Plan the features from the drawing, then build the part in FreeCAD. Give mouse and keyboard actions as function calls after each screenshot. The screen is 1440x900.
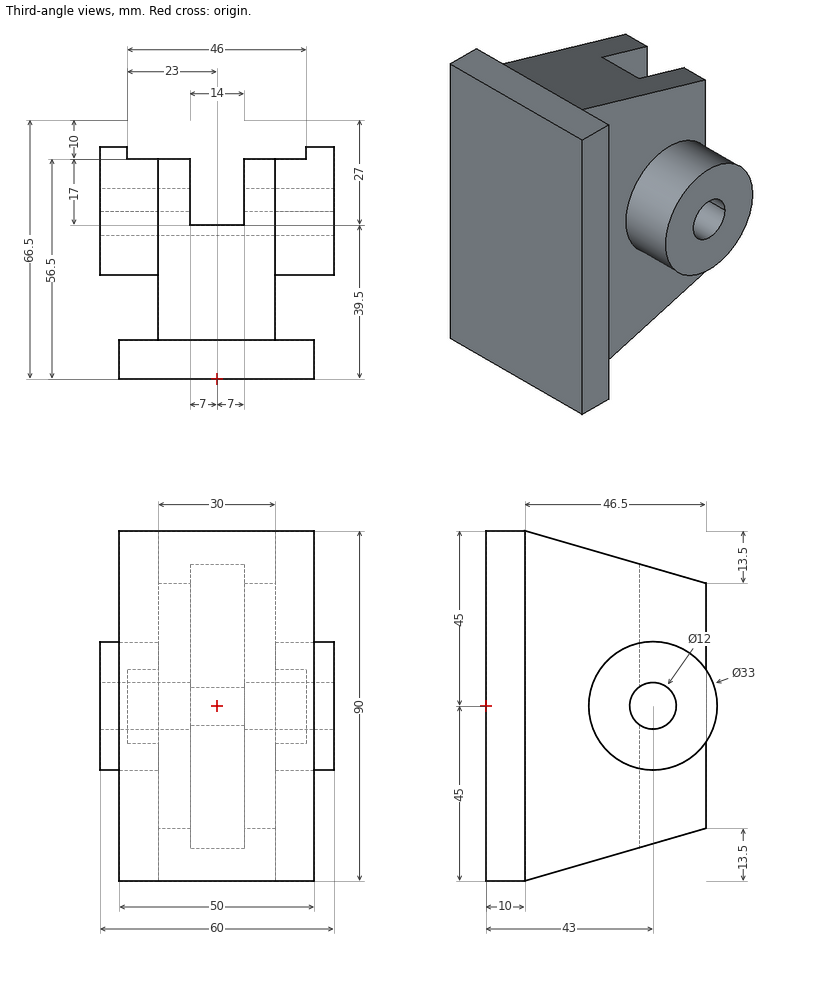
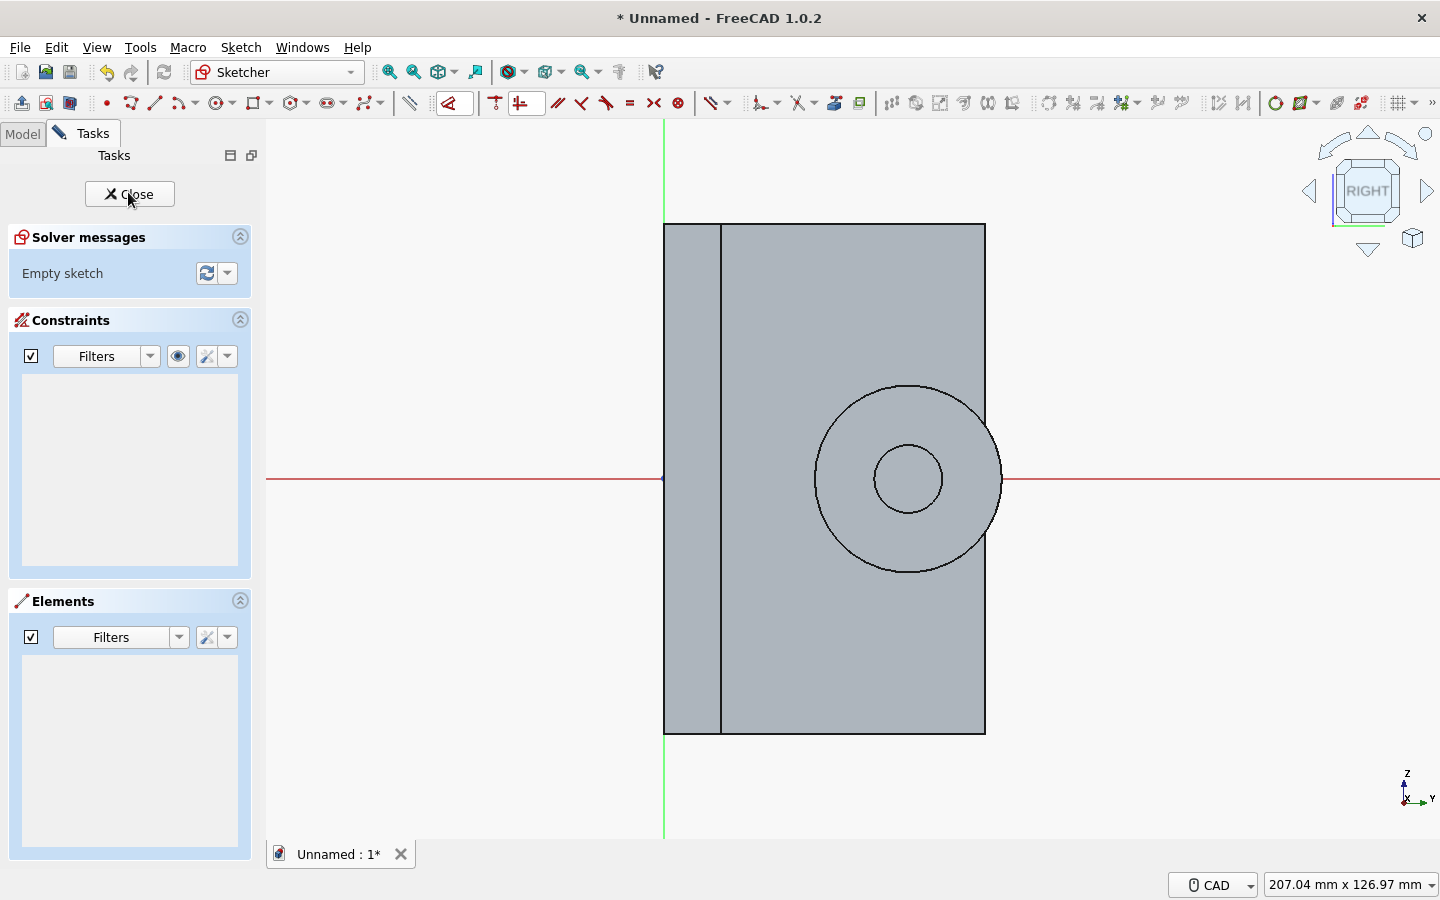
click(70, 104)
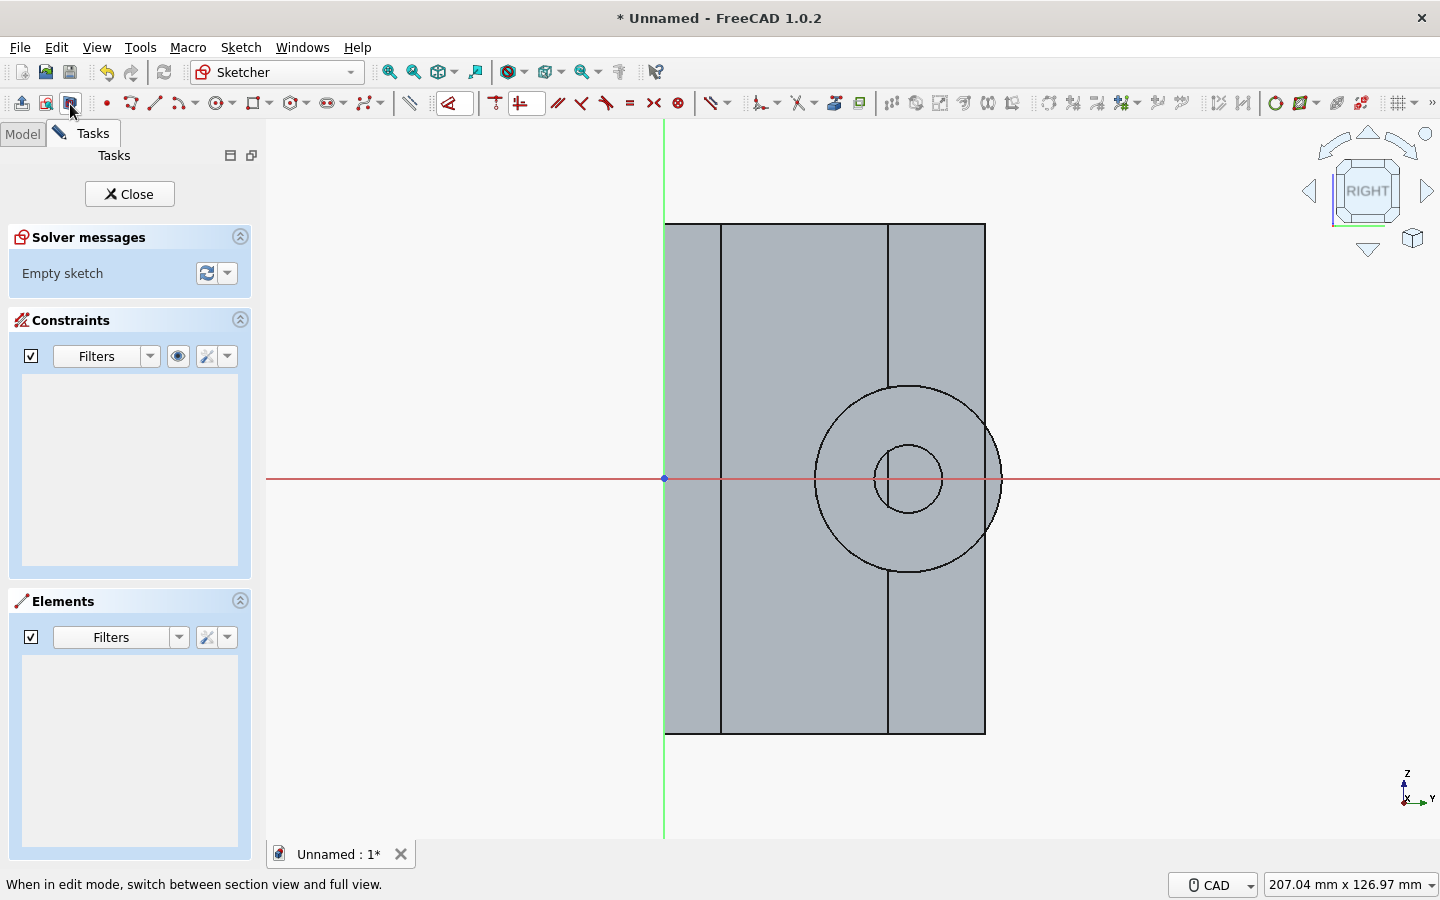
click(132, 104)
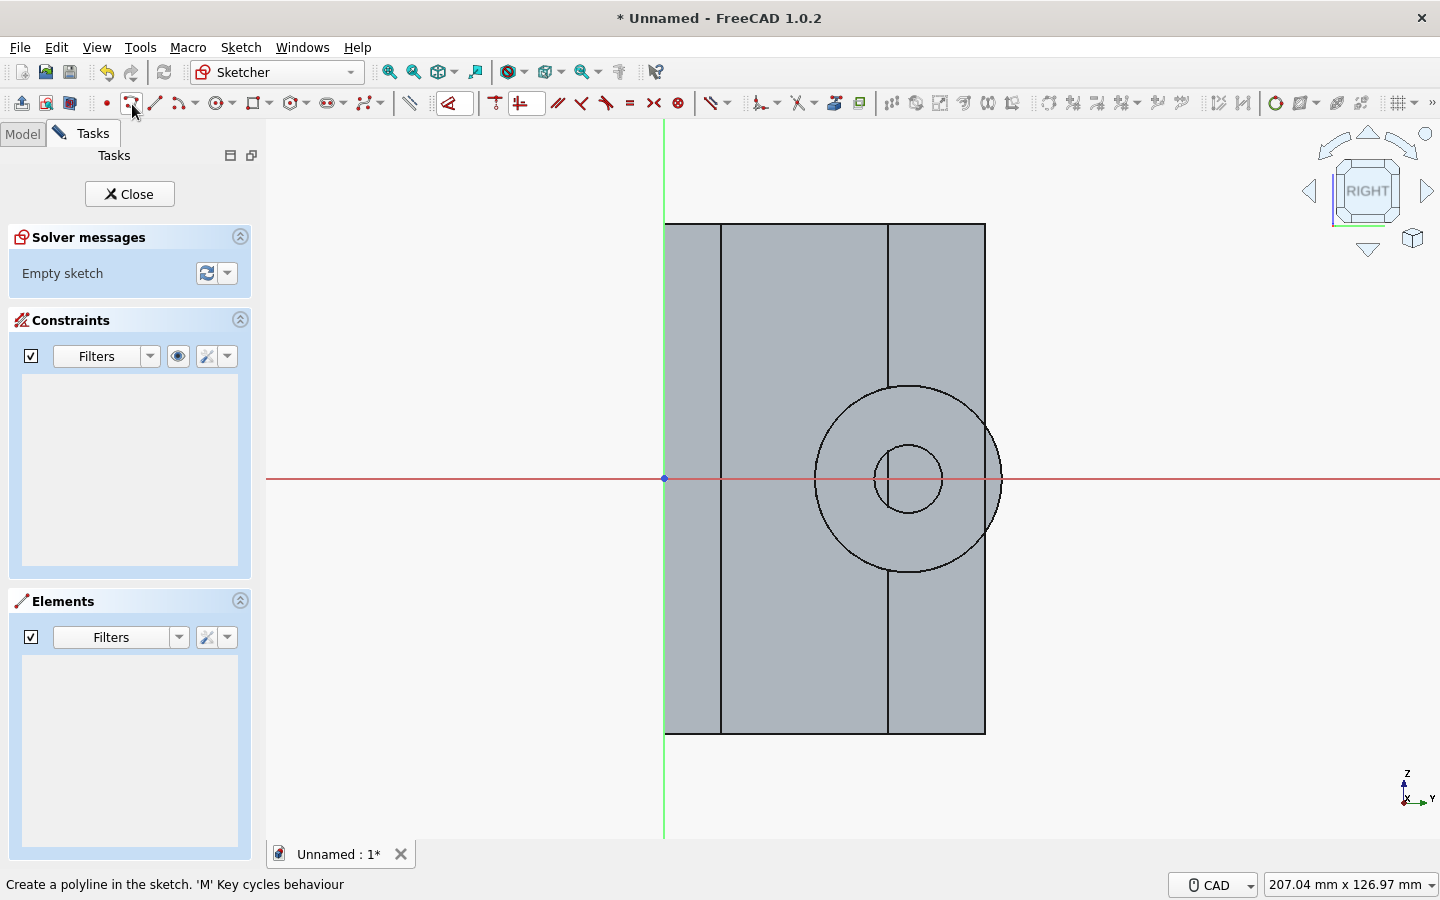
click(721, 224)
click(985, 300)
click(985, 224)
click(721, 225)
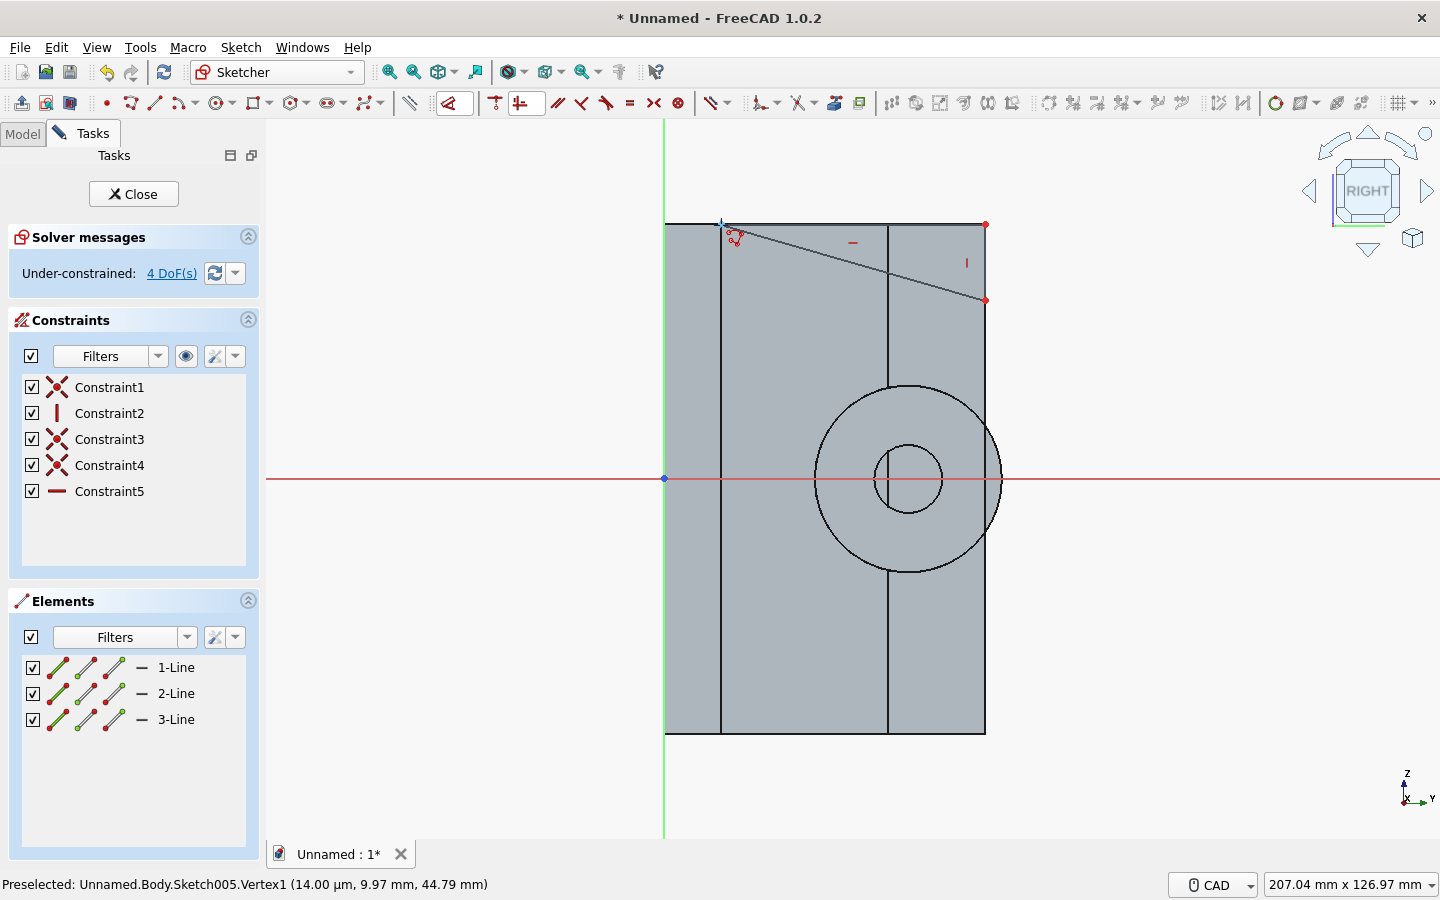
click(721, 734)
click(985, 734)
click(985, 658)
click(721, 735)
key(Escape)
key(Escape)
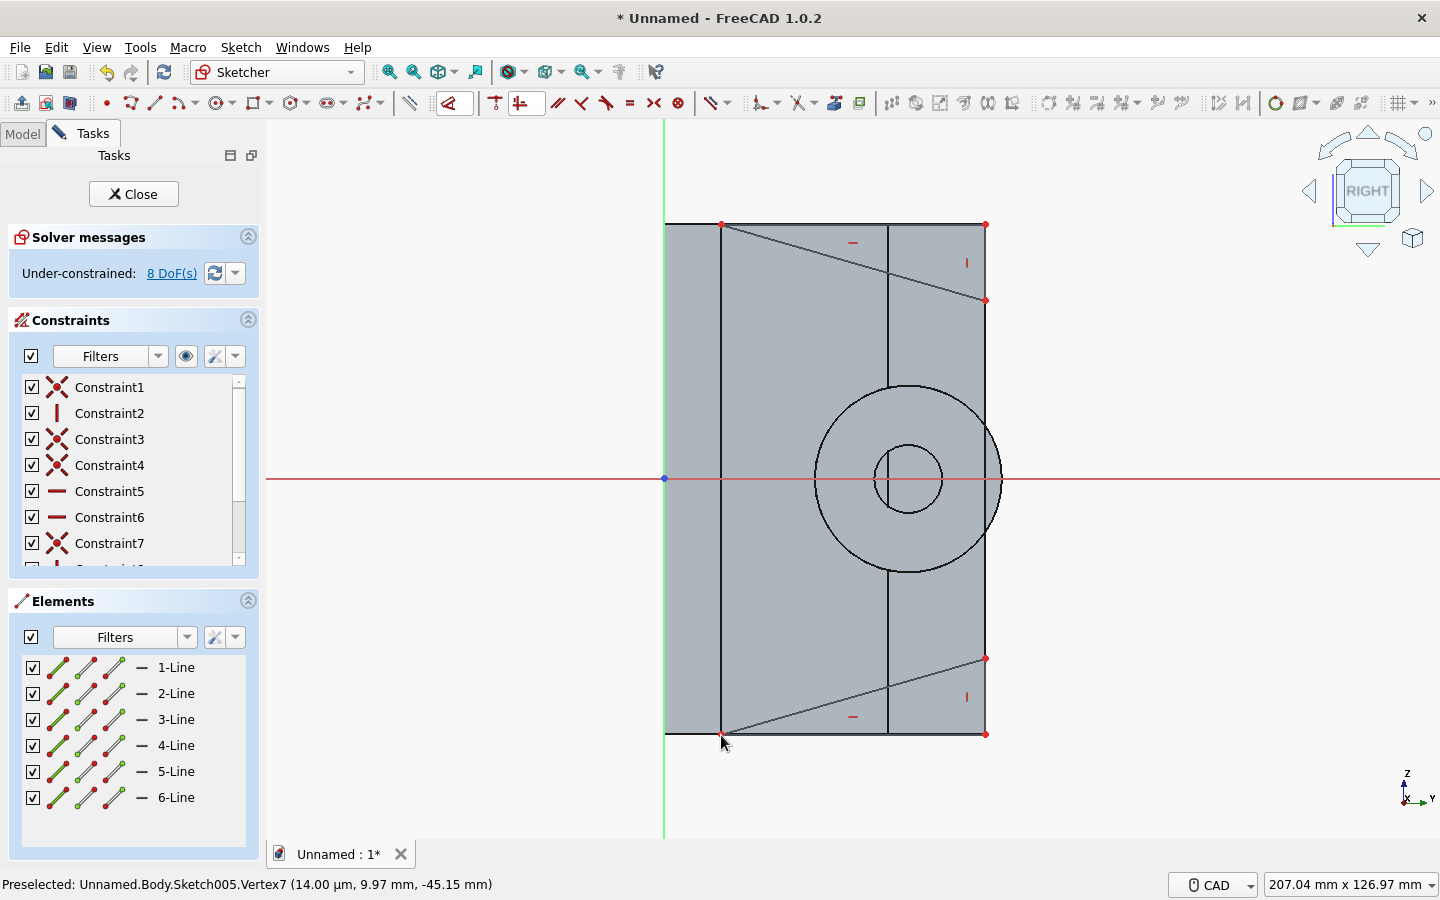
click(721, 225)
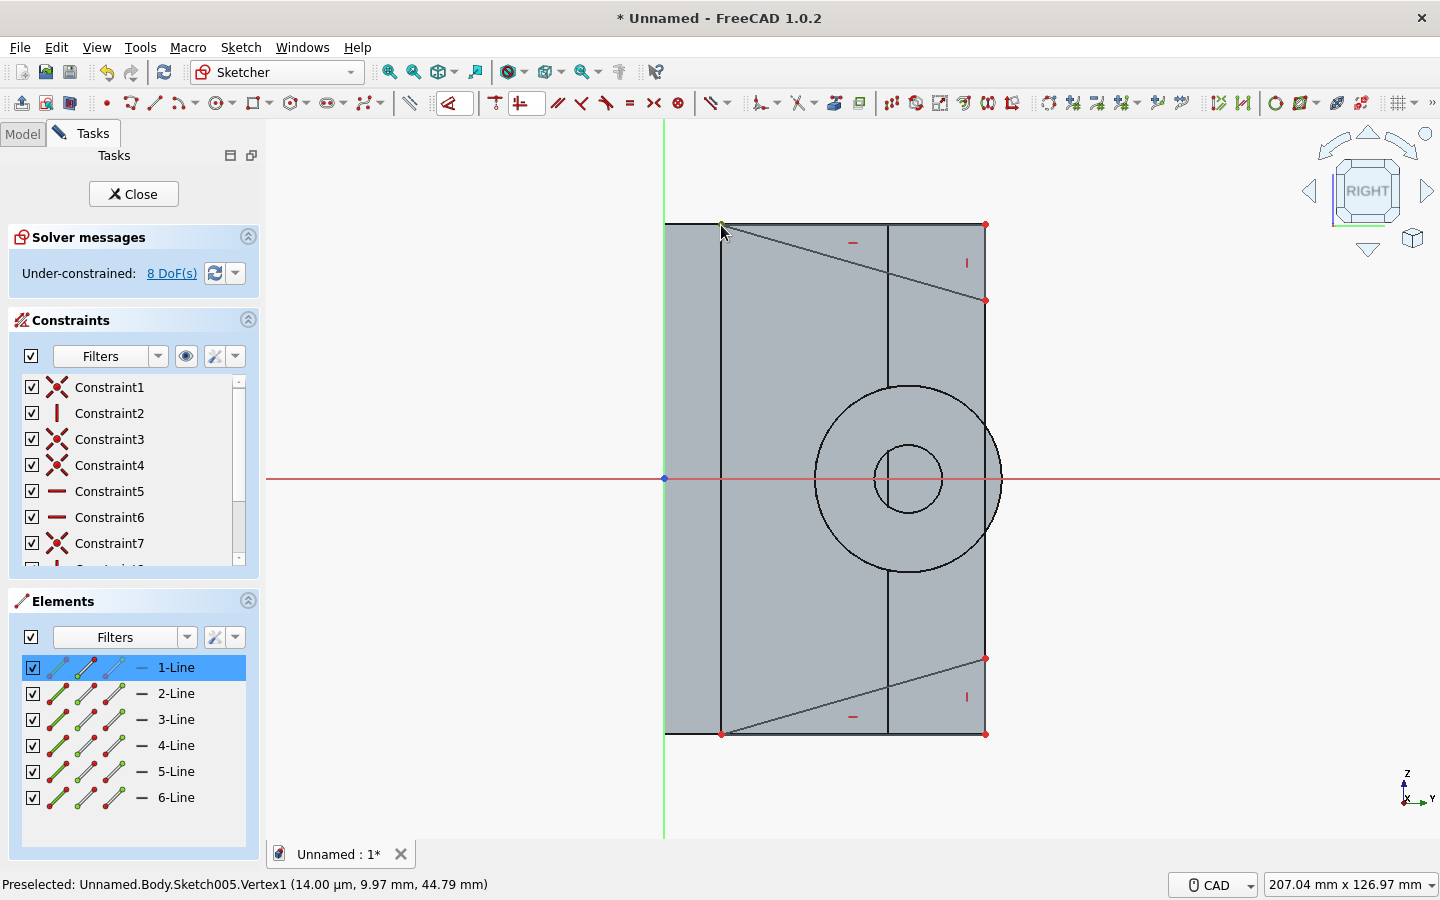
click(468, 104)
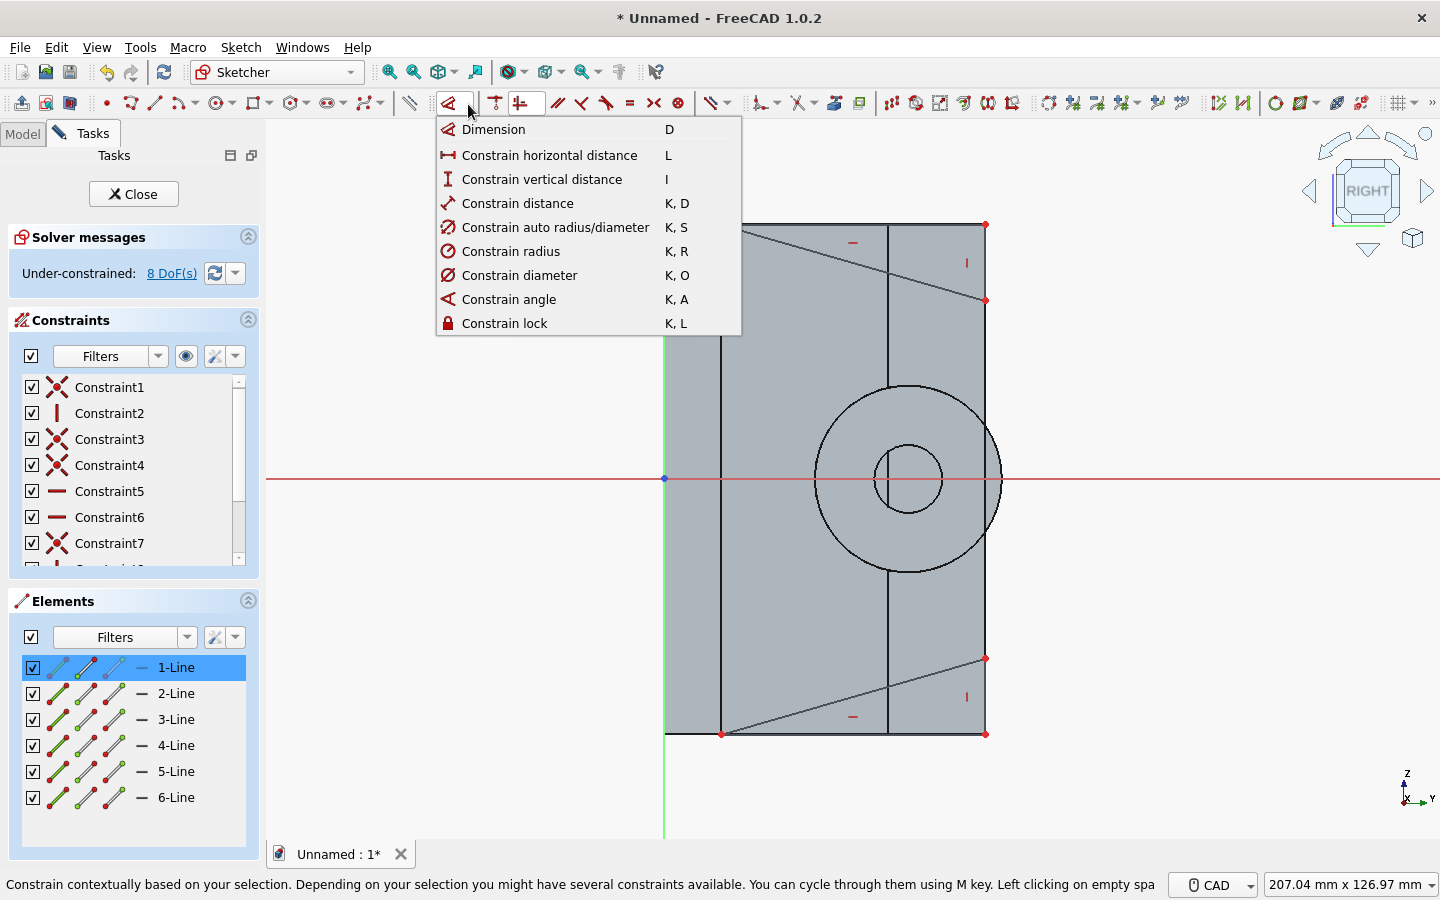
click(589, 155)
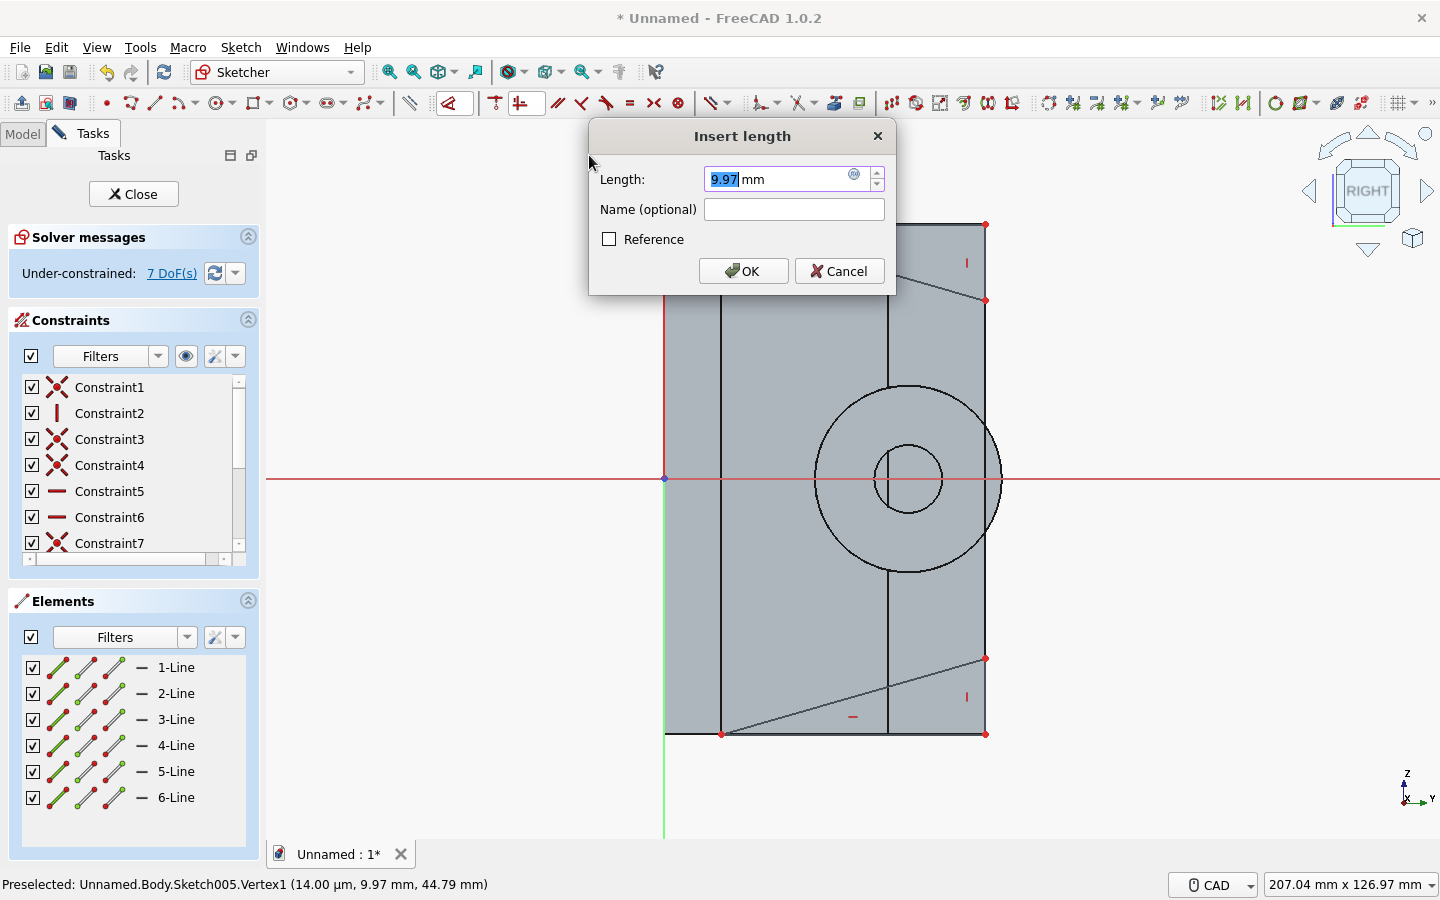
text(10)
key(Return)